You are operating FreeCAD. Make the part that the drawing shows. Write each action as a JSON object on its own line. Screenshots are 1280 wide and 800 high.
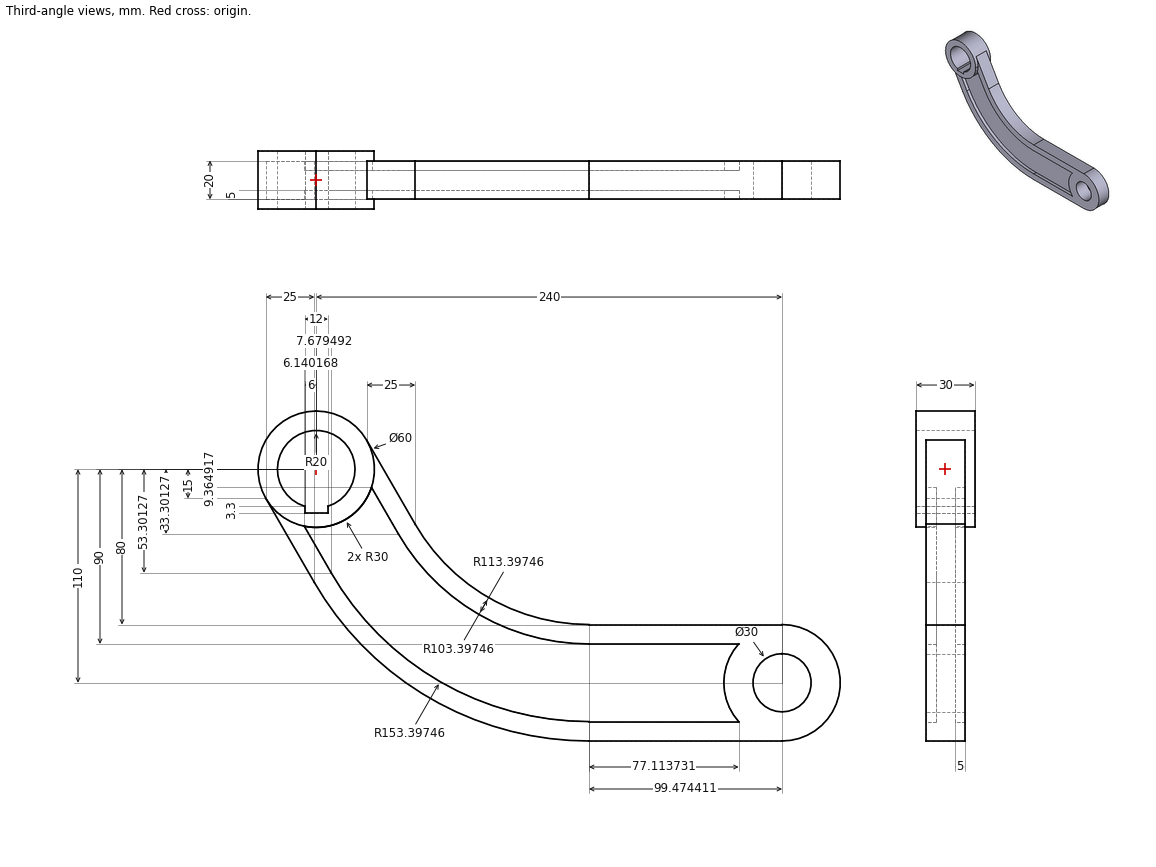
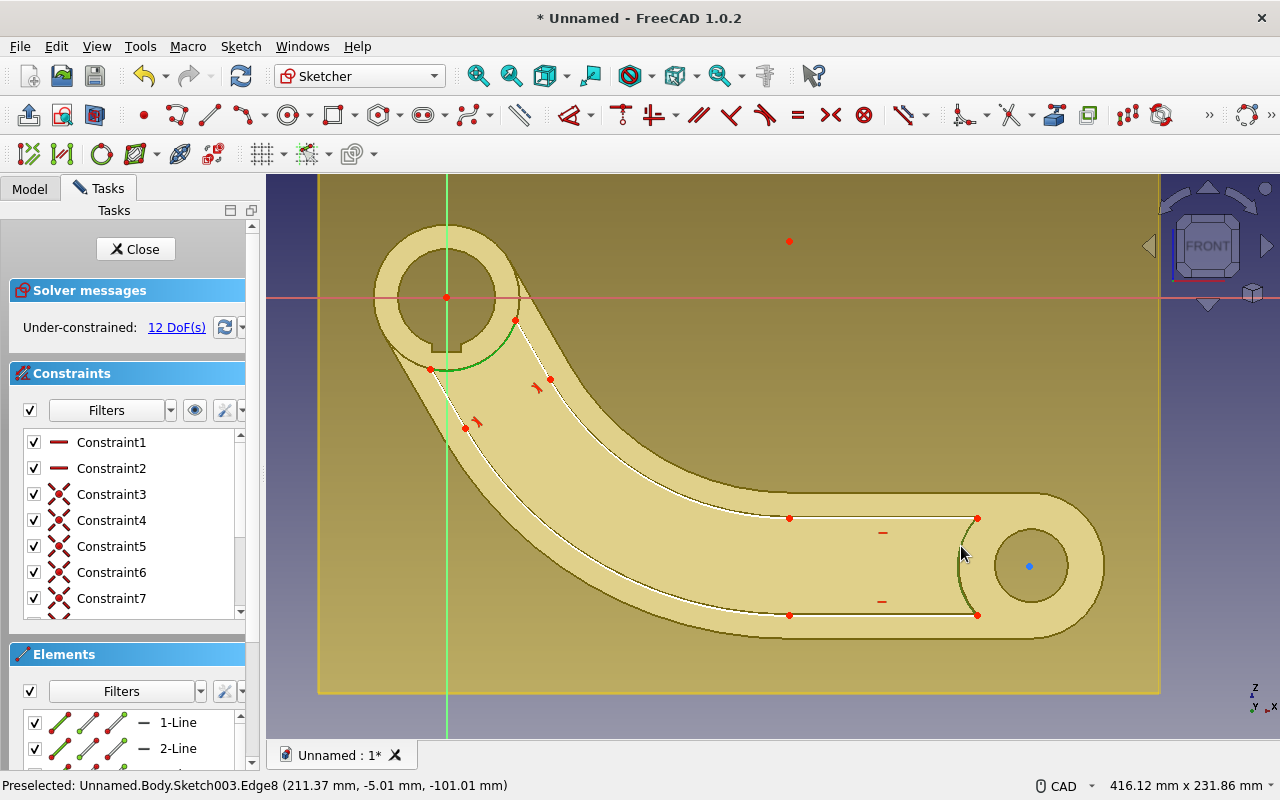
{"action": "left_click", "coordinate": [798, 116]}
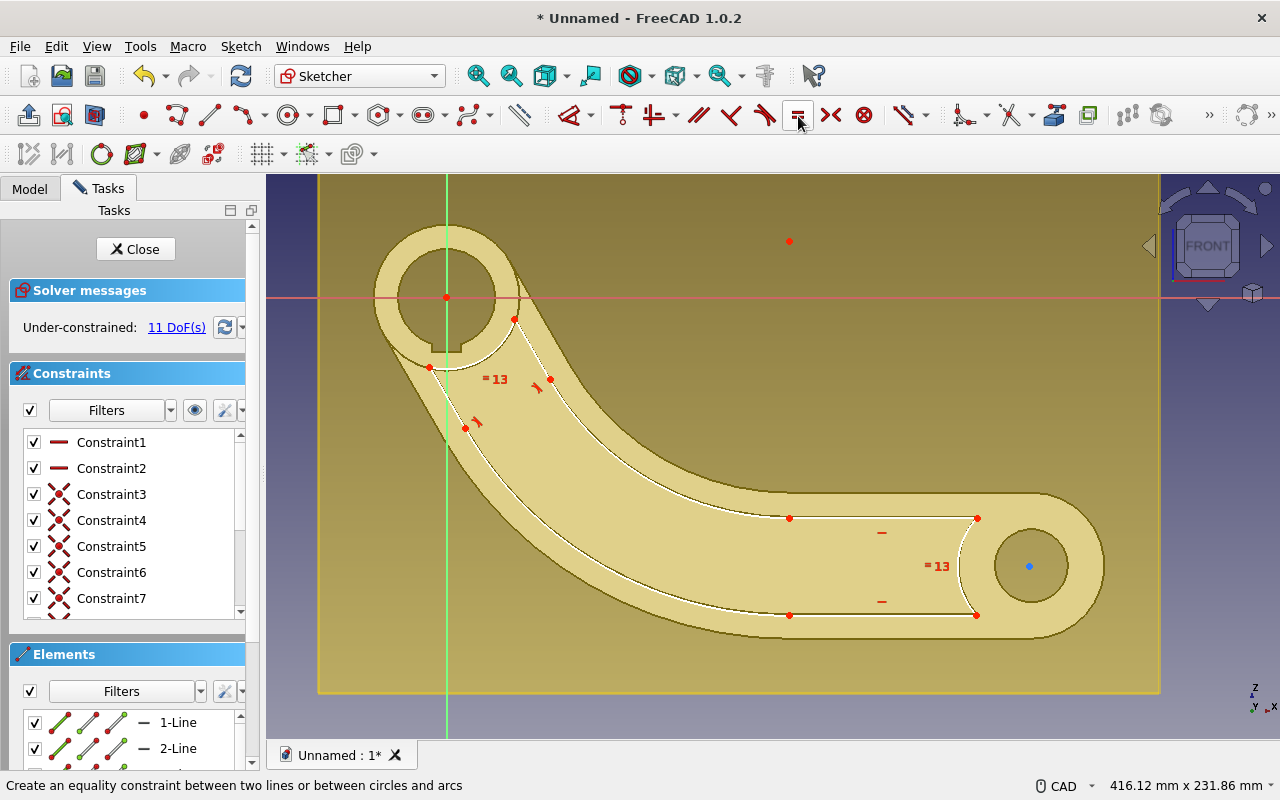
{"action": "left_click", "coordinate": [568, 116]}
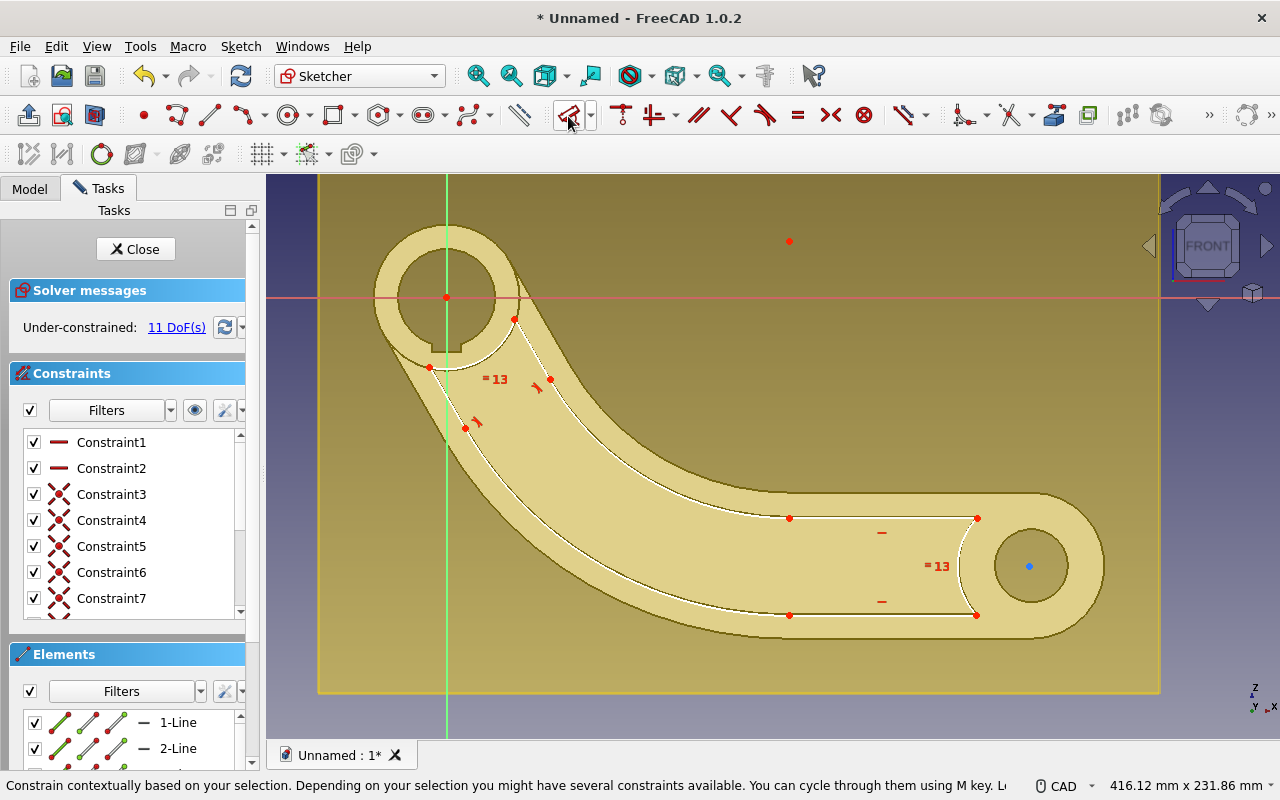
{"action": "left_click", "coordinate": [604, 447]}
{"action": "left_click", "coordinate": [583, 471]}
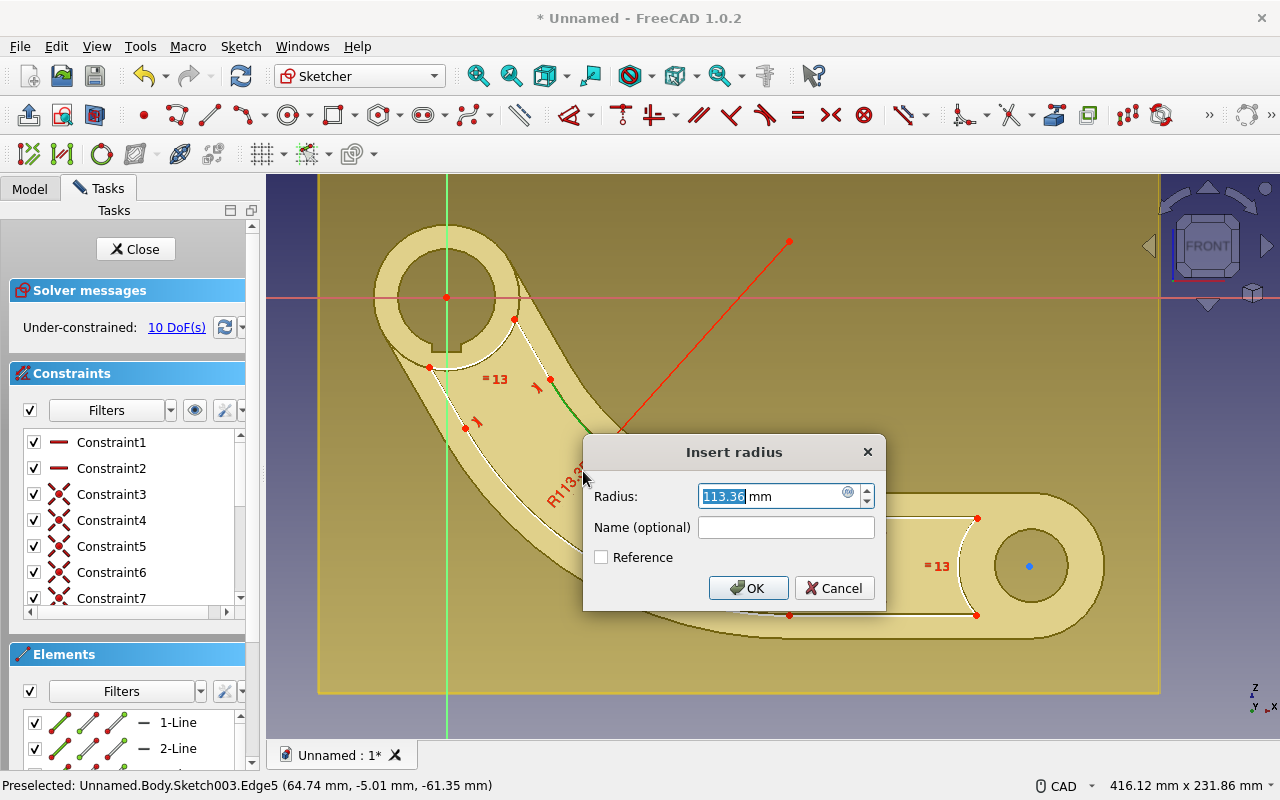
{"action": "type", "text": "113.39746"}
{"action": "key", "text": "Return"}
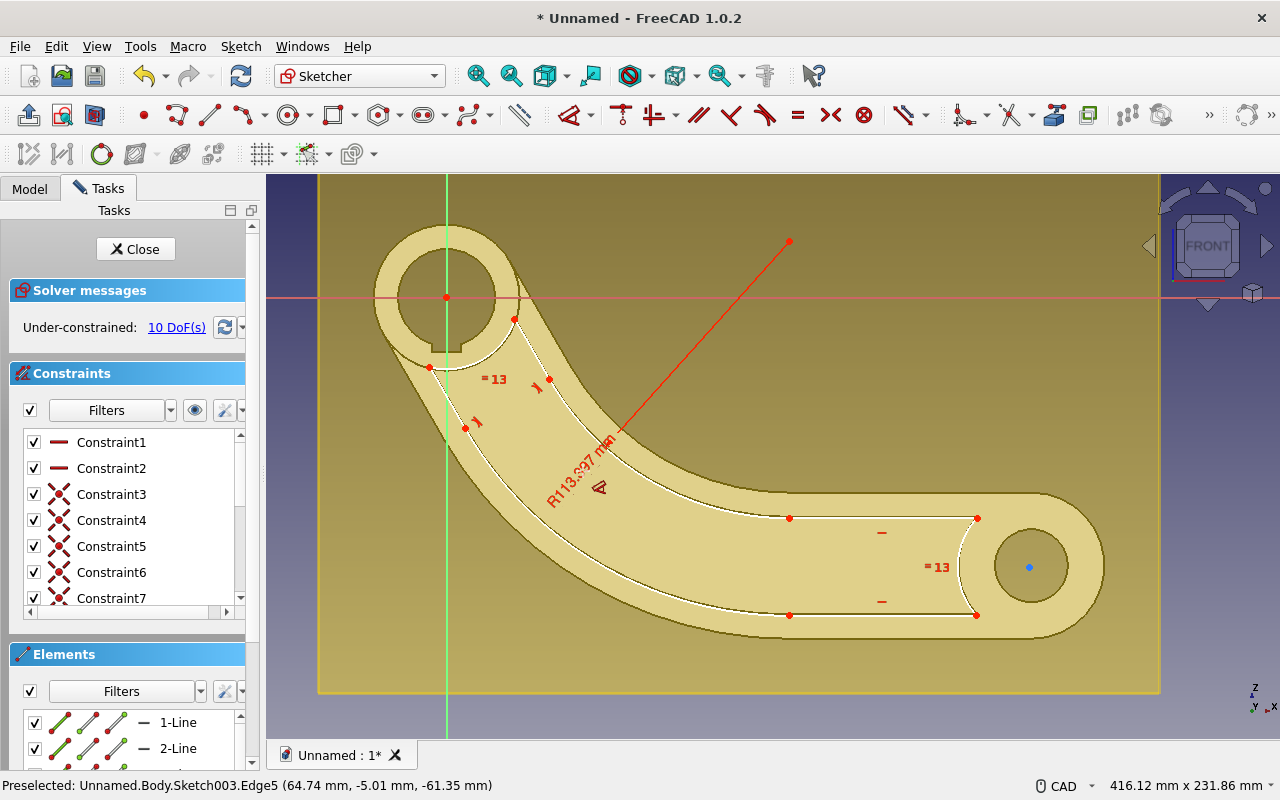
{"action": "left_click", "coordinate": [462, 368]}
{"action": "left_click", "coordinate": [469, 399]}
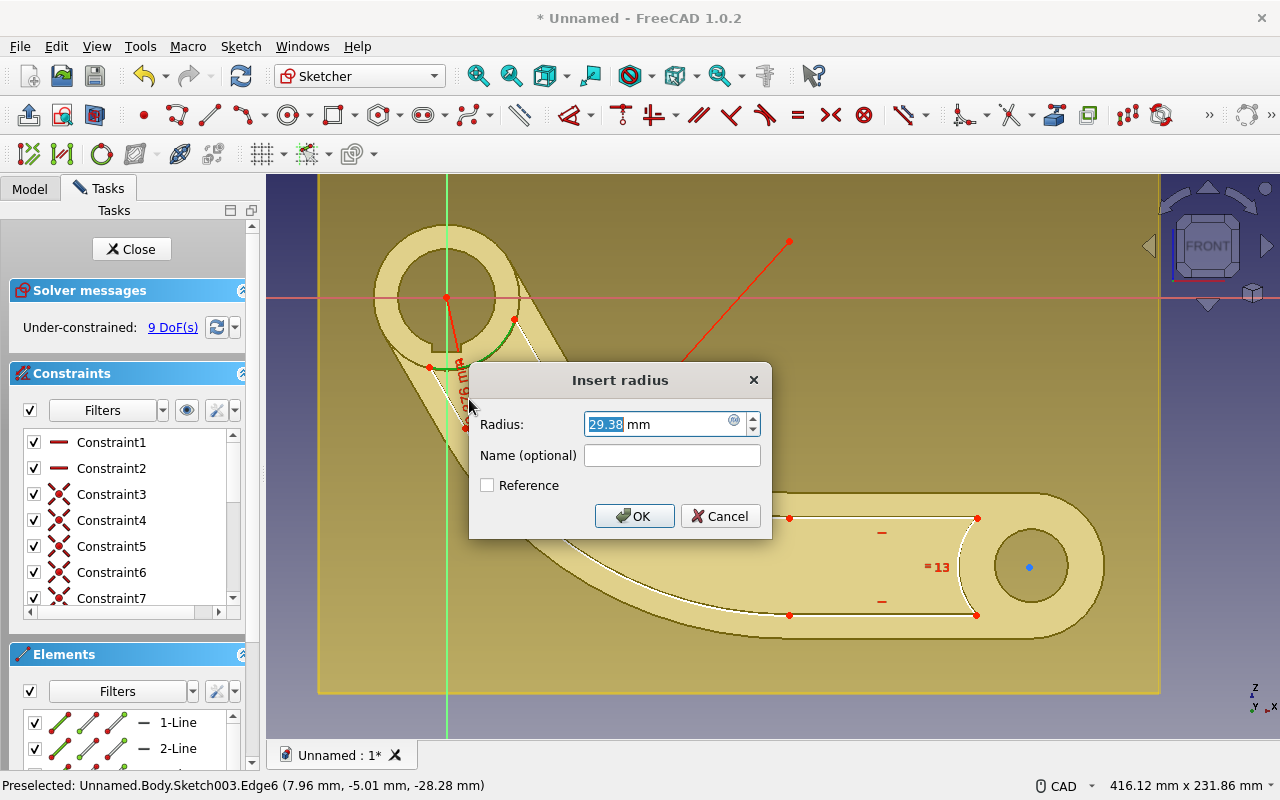
{"action": "type", "text": "30"}
{"action": "key", "text": "Return"}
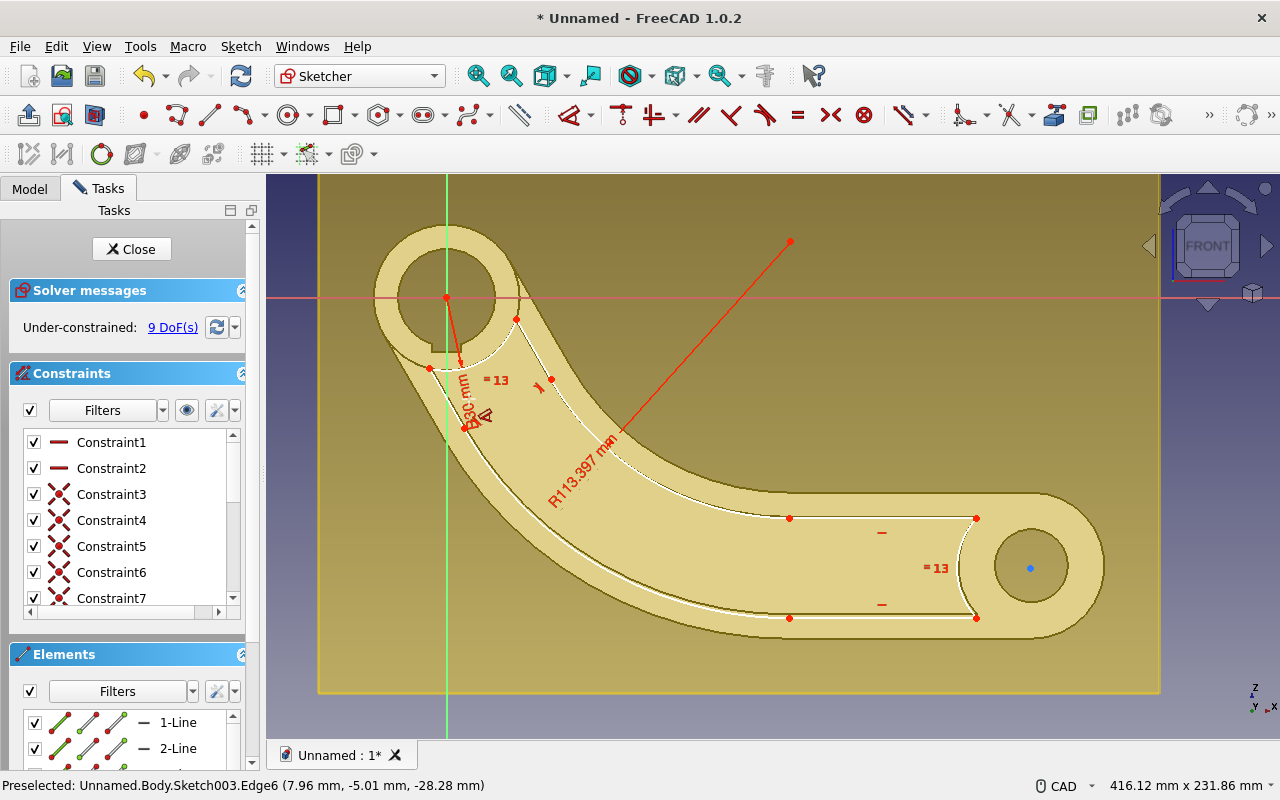
{"action": "left_click", "coordinate": [538, 521]}
{"action": "left_click", "coordinate": [517, 545]}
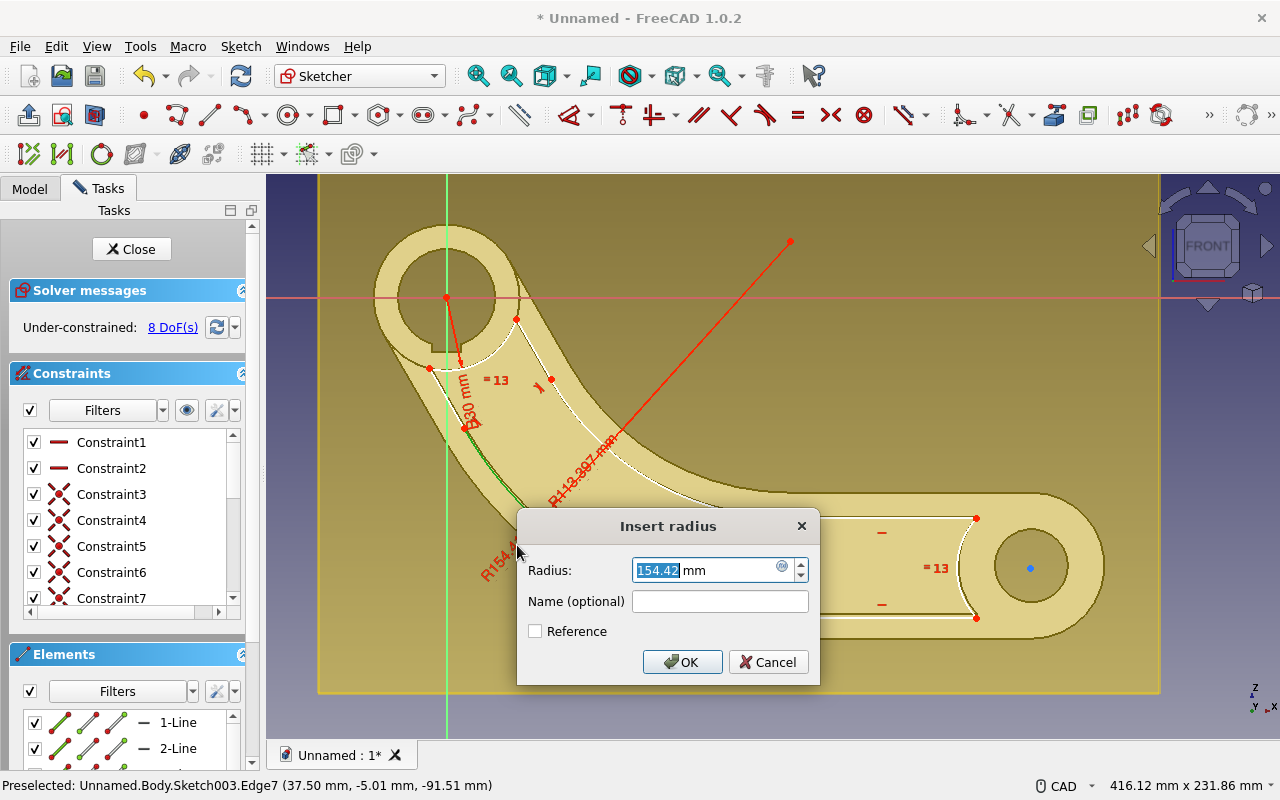
{"action": "type", "text": "153.39746"}
{"action": "key", "text": "Return"}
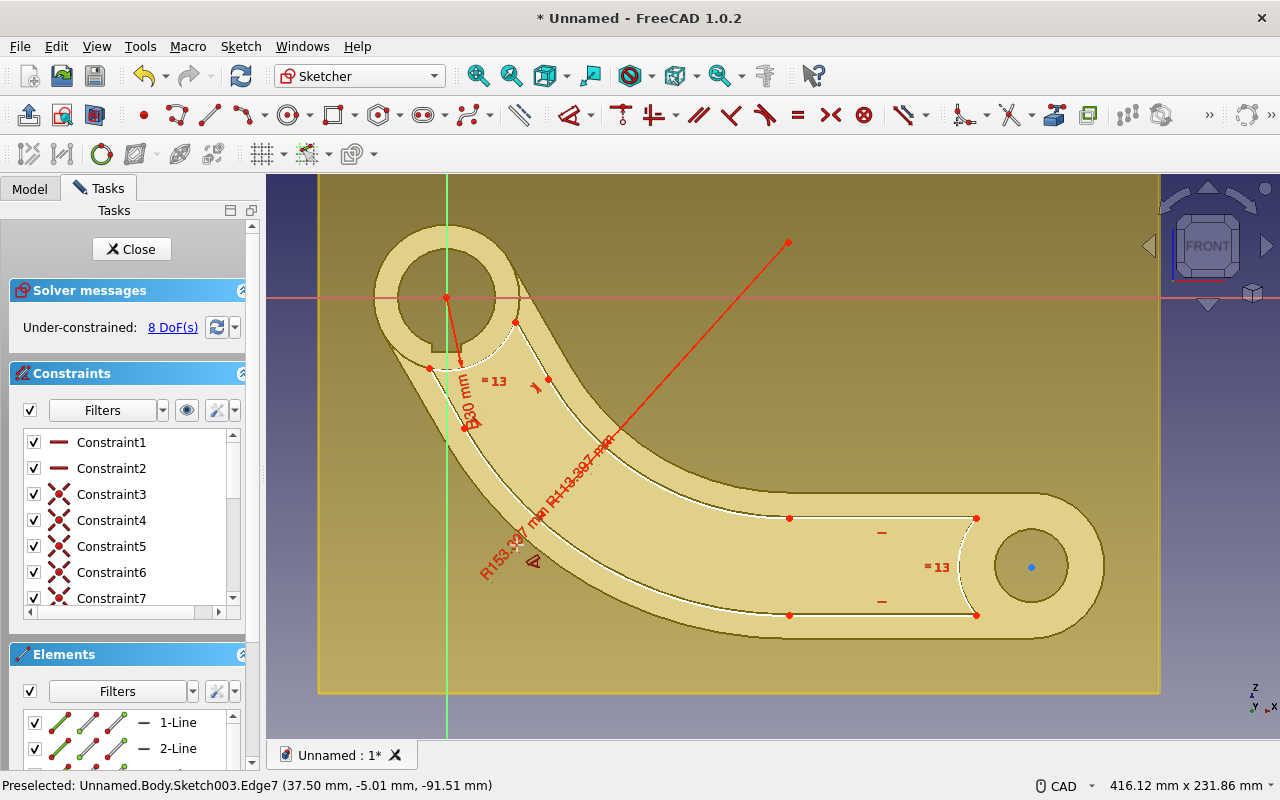
{"action": "left_click", "coordinate": [977, 518]}
{"action": "left_click", "coordinate": [1011, 408]}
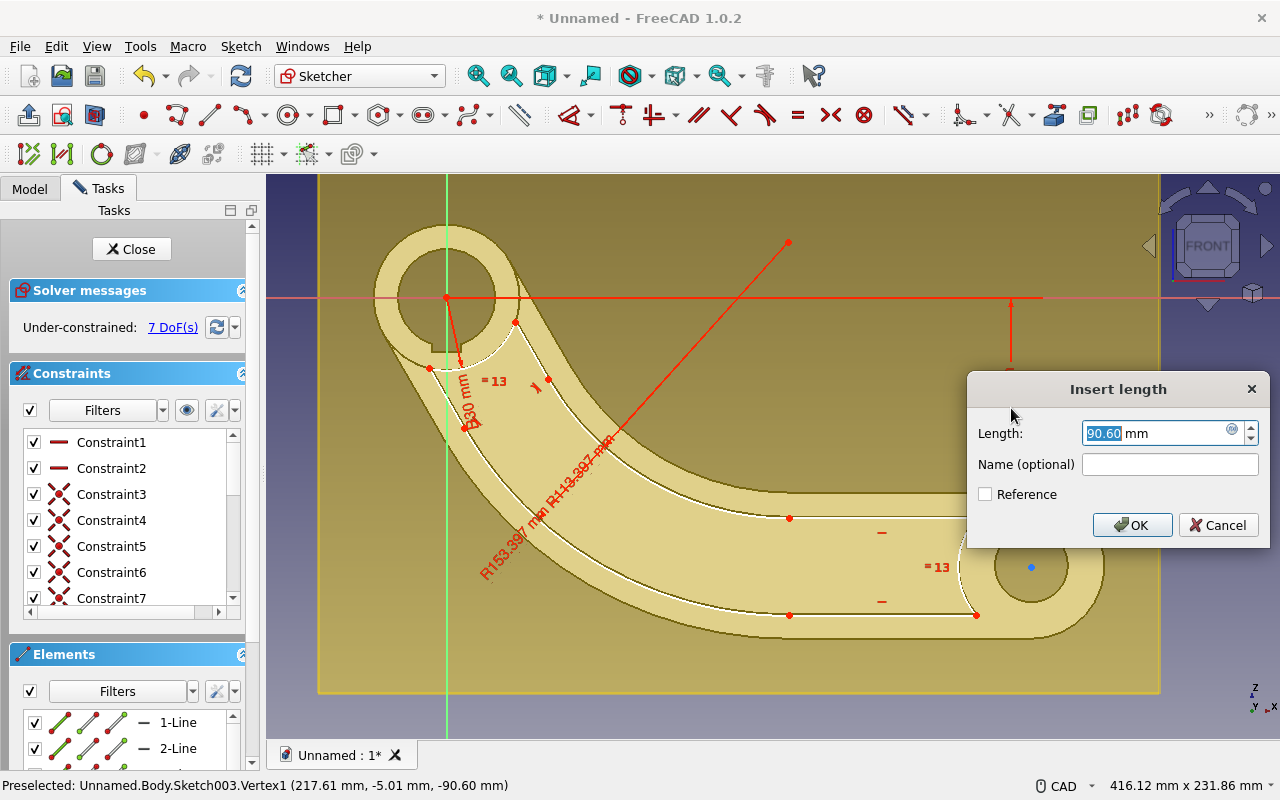
{"action": "type", "text": "90"}
{"action": "key", "text": "Return"}